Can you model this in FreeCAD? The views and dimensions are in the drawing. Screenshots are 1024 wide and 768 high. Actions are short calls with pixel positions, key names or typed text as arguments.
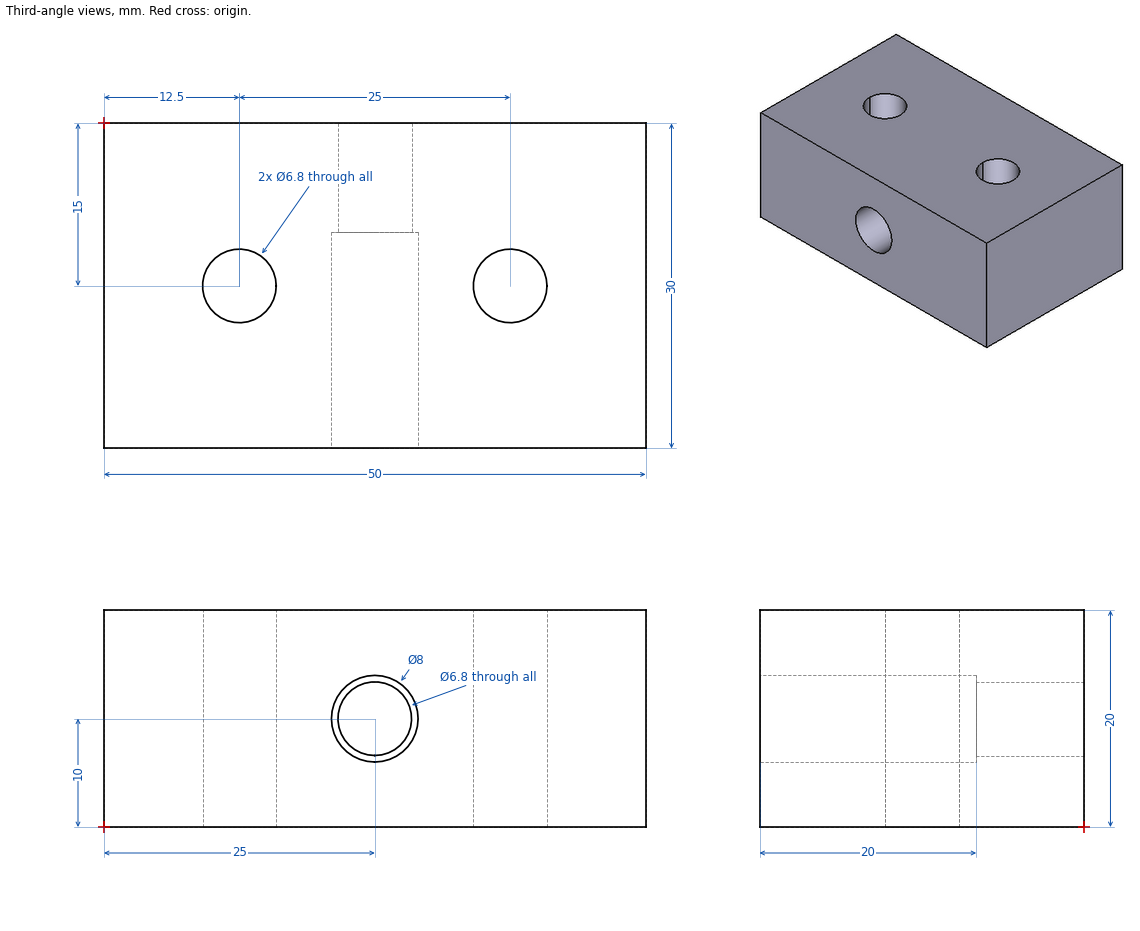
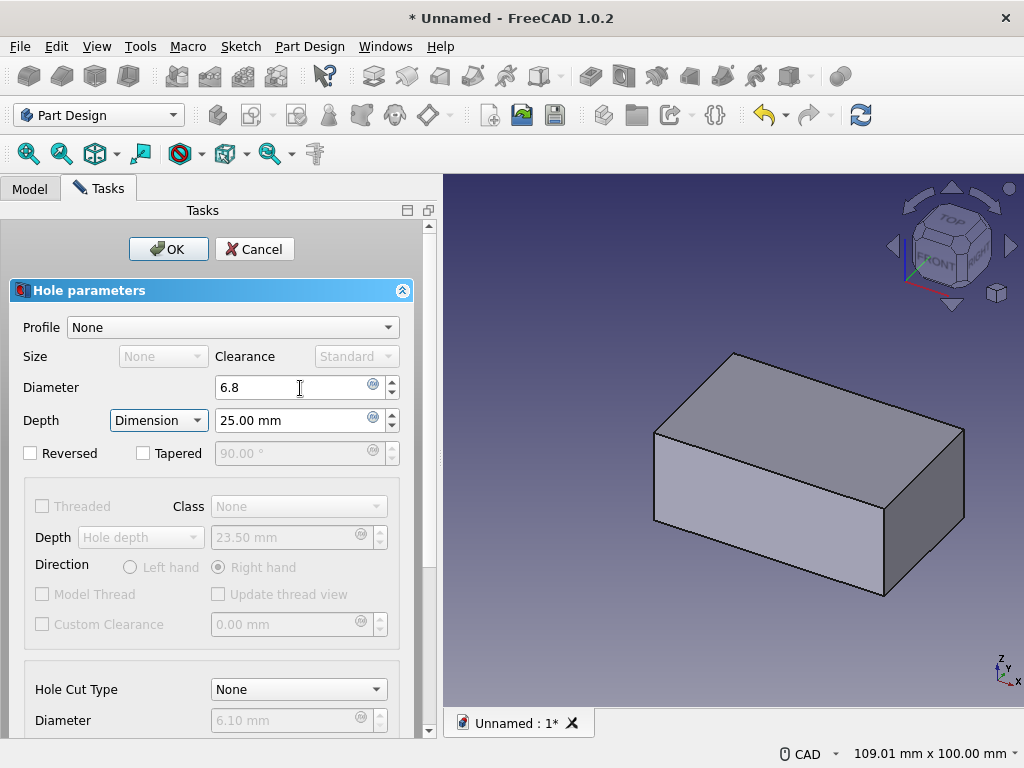
click(160, 420)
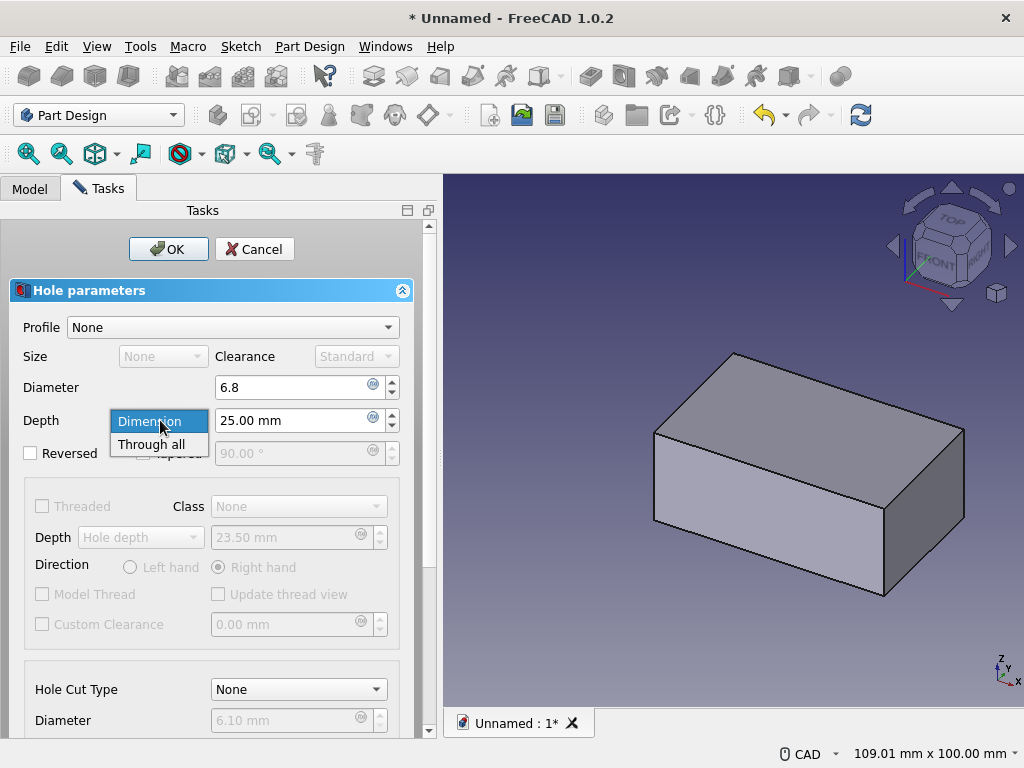
click(158, 444)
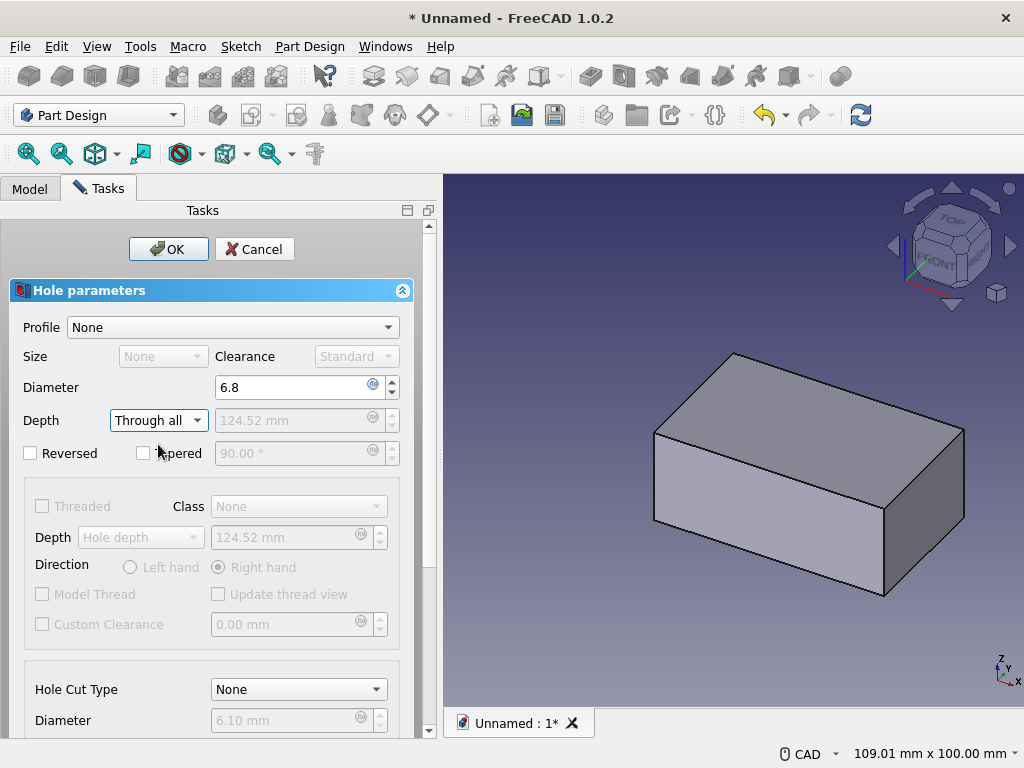
click(31, 453)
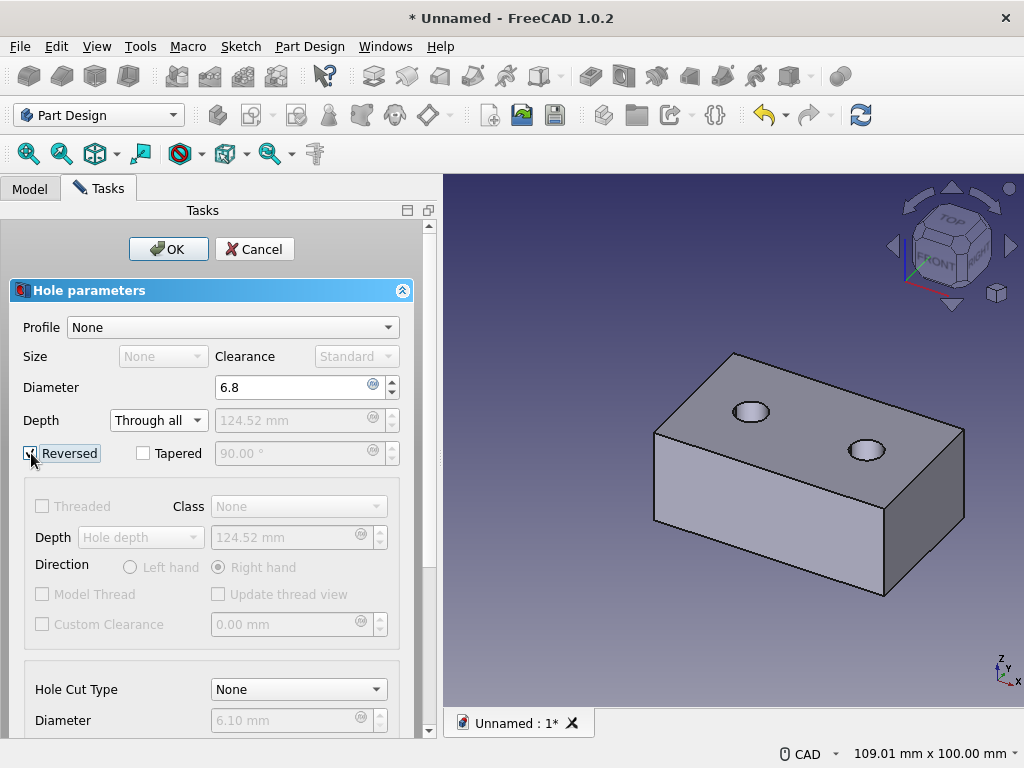
click(169, 249)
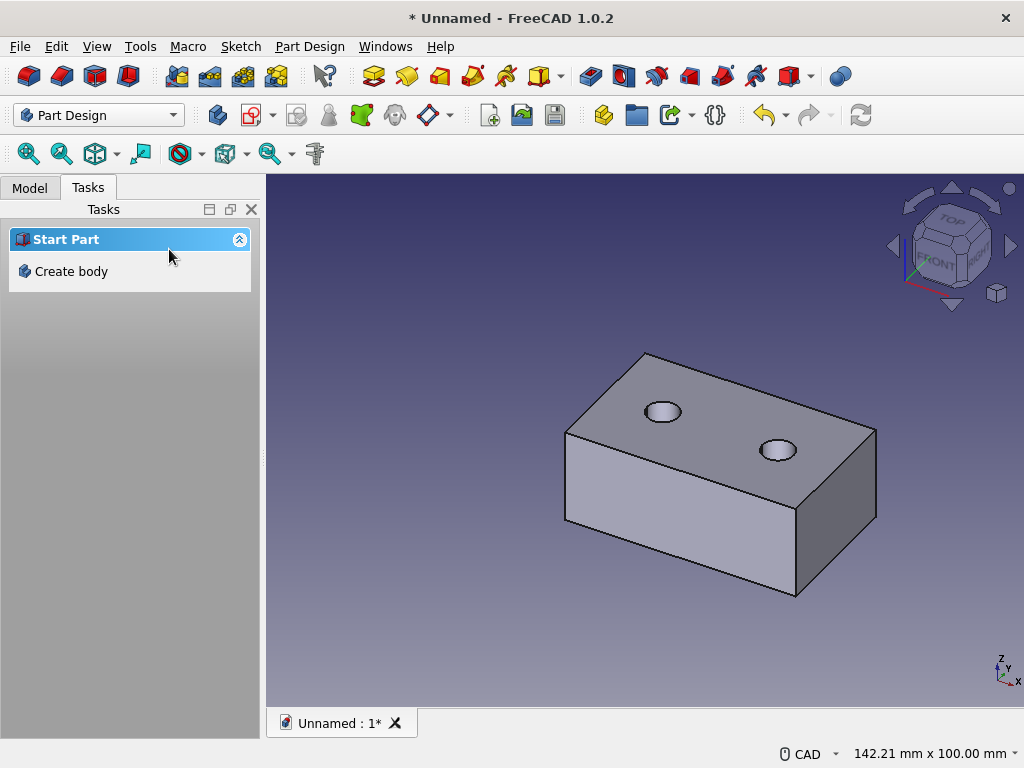
key(4)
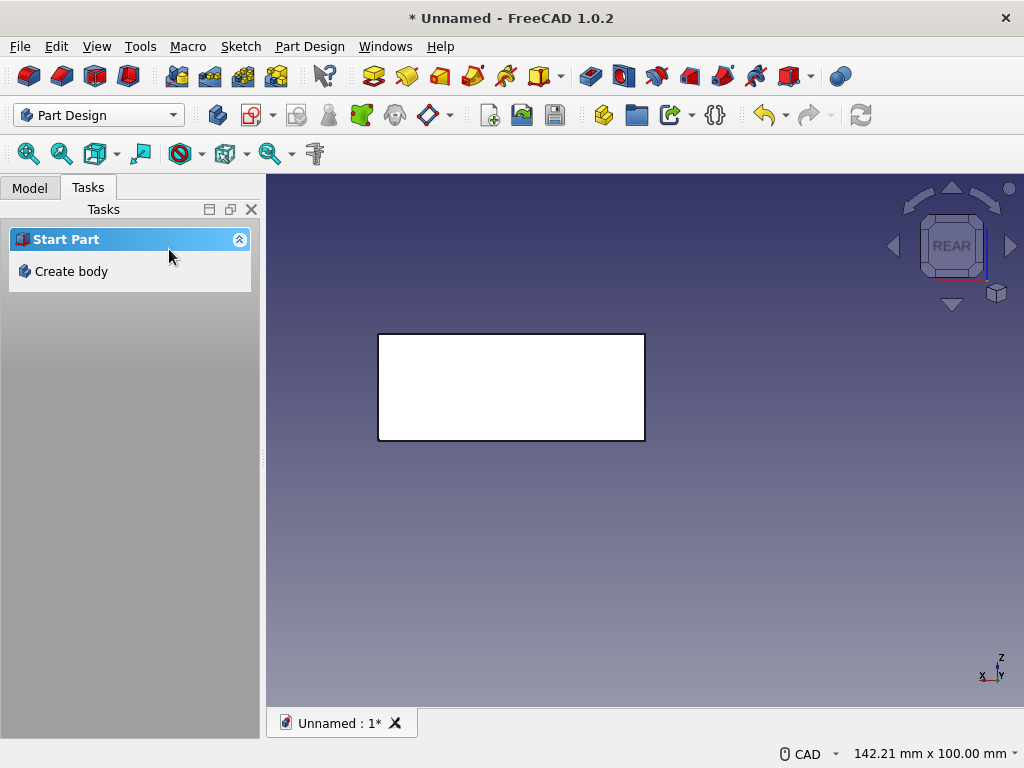
click(29, 154)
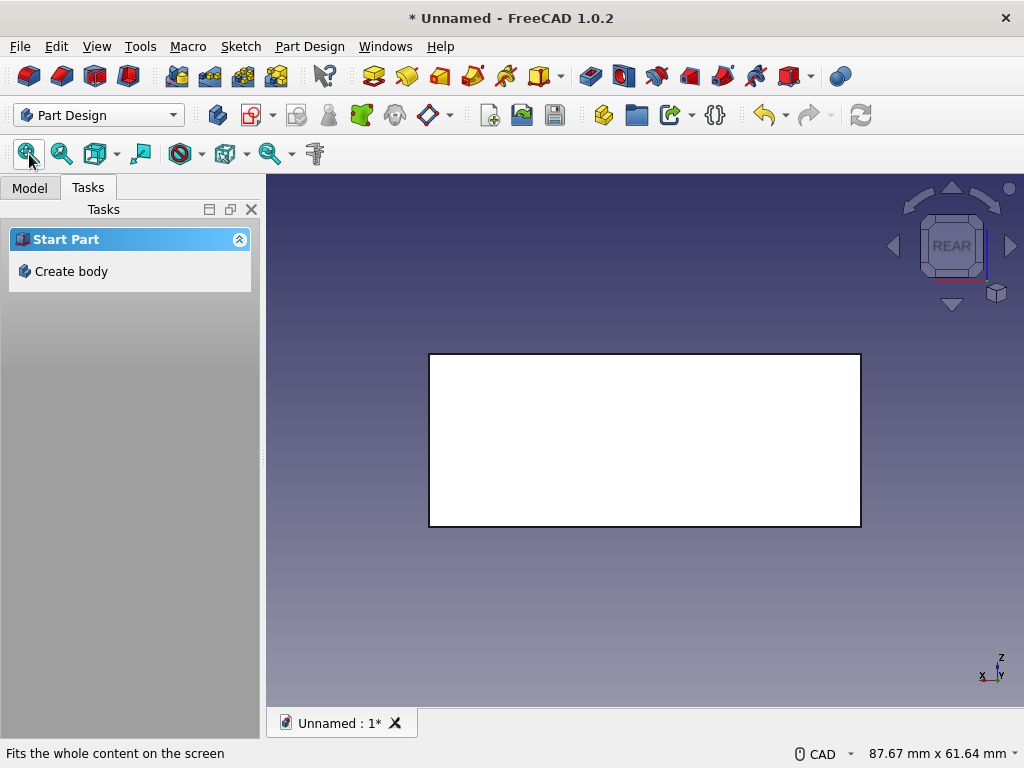
click(521, 440)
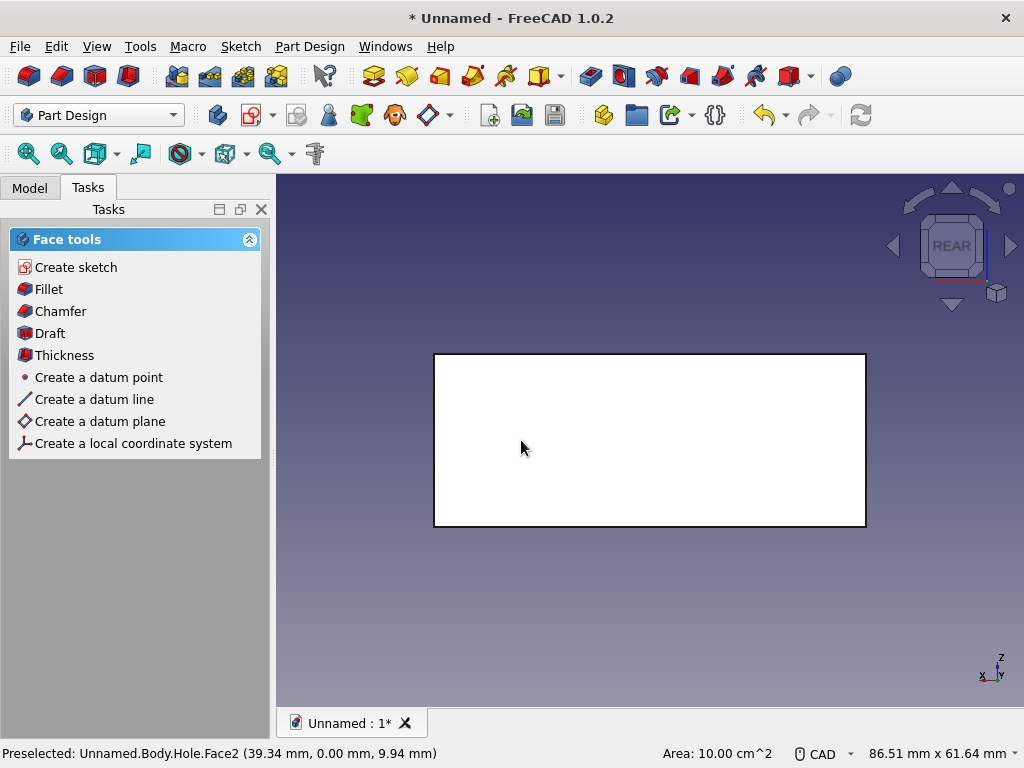
click(250, 116)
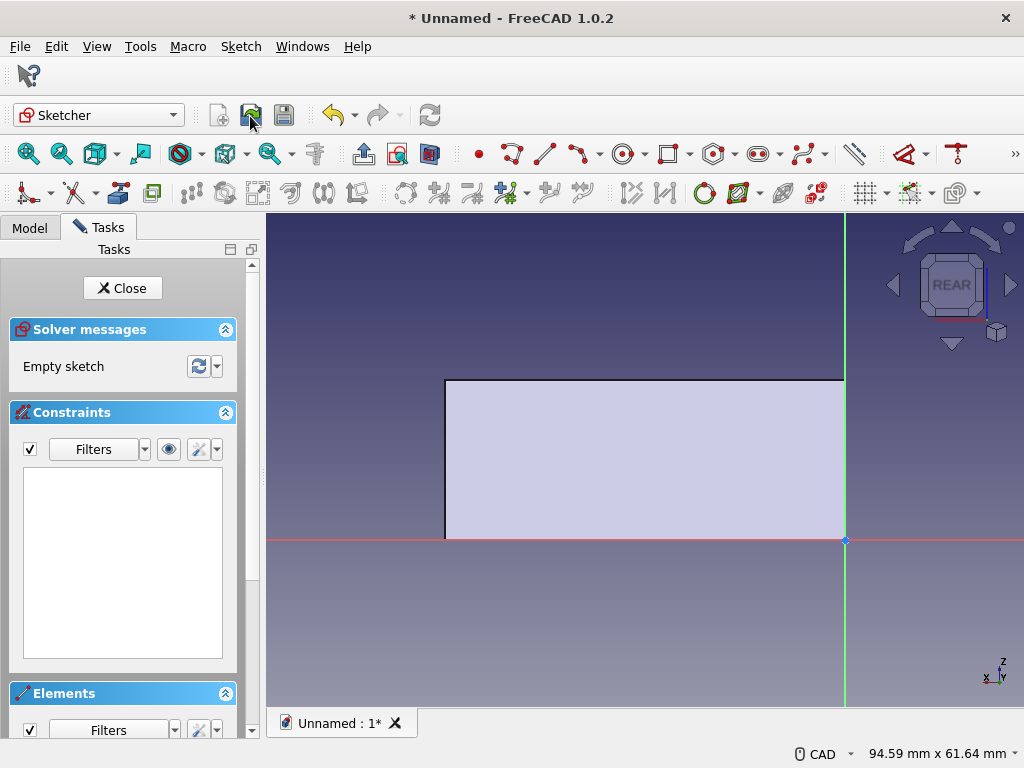
scroll(659, 460, up, 9)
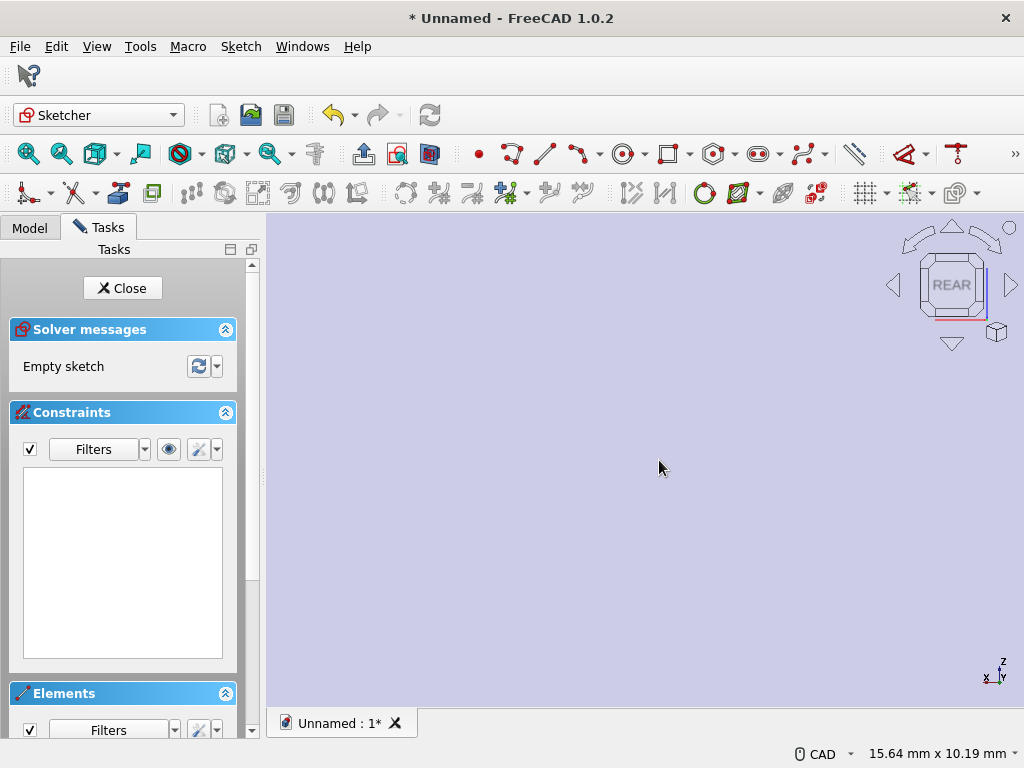
click(622, 154)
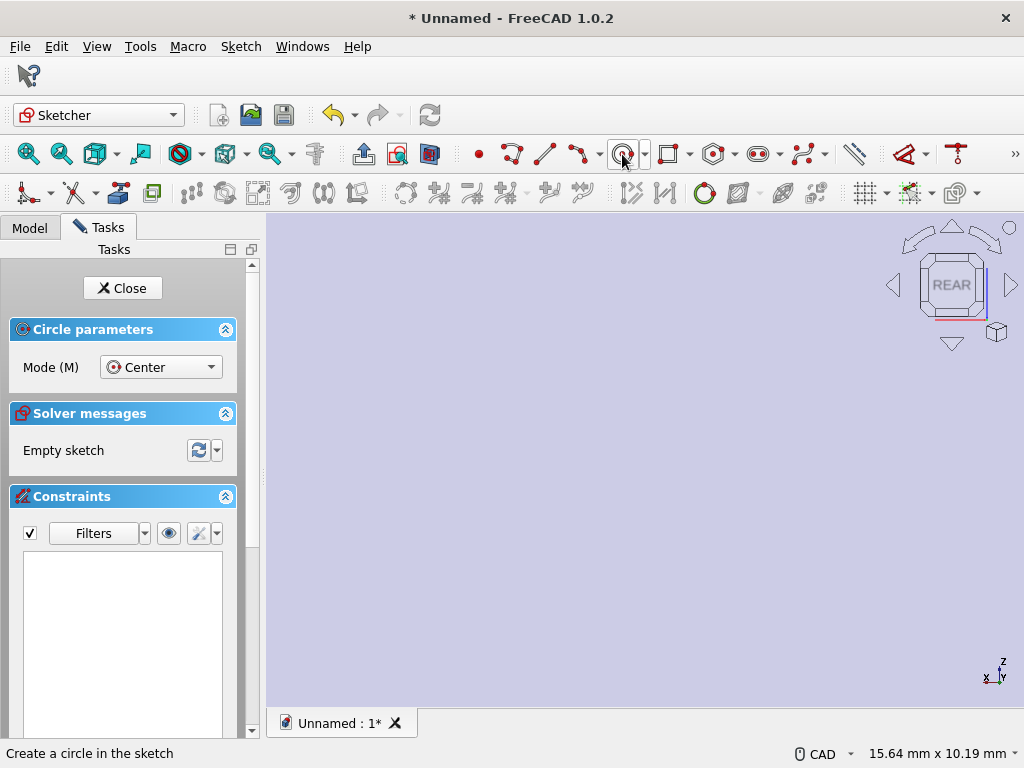
click(572, 457)
move(688, 341)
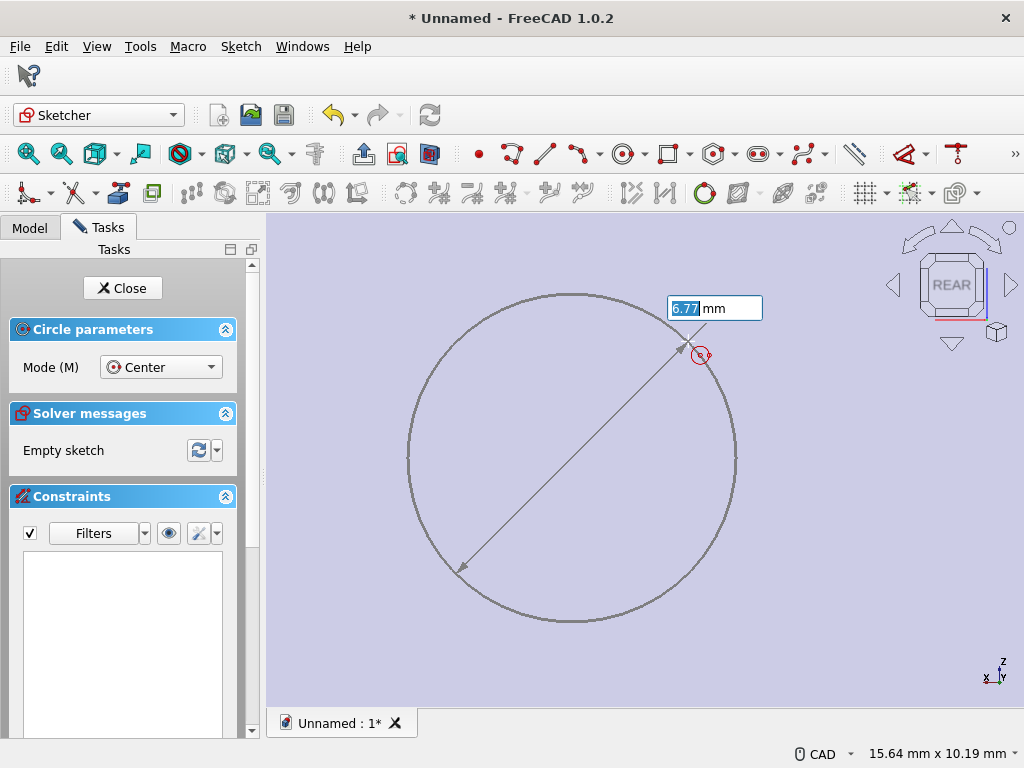
text(6.8)
key(Return)
key(Escape)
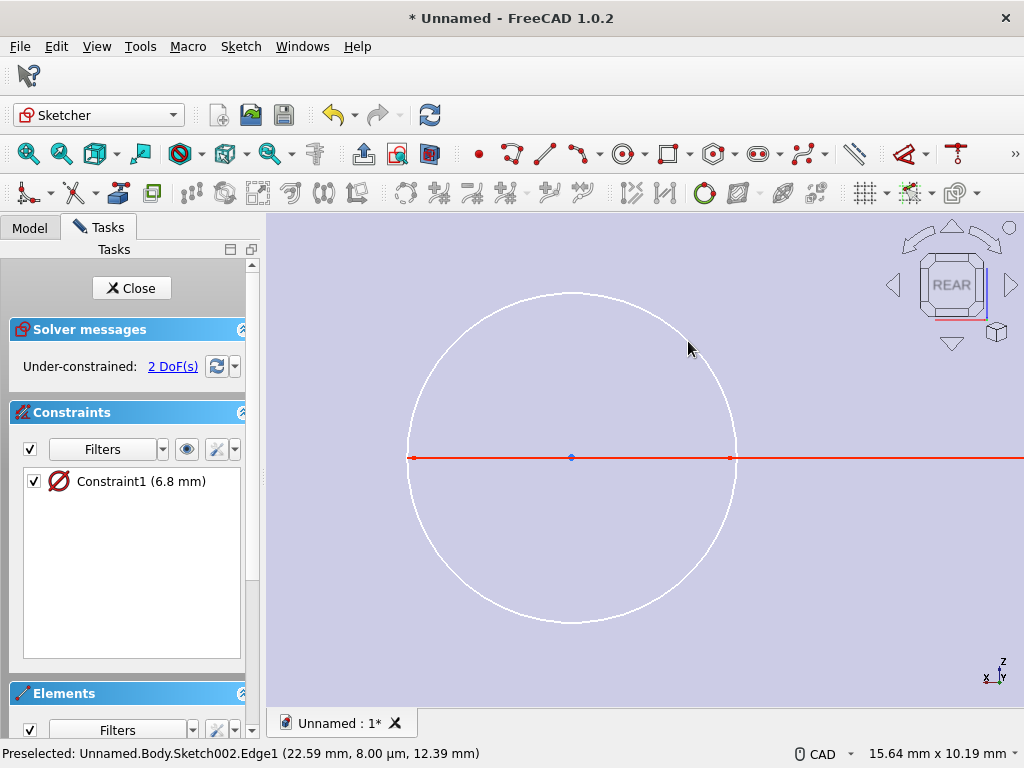
click(904, 154)